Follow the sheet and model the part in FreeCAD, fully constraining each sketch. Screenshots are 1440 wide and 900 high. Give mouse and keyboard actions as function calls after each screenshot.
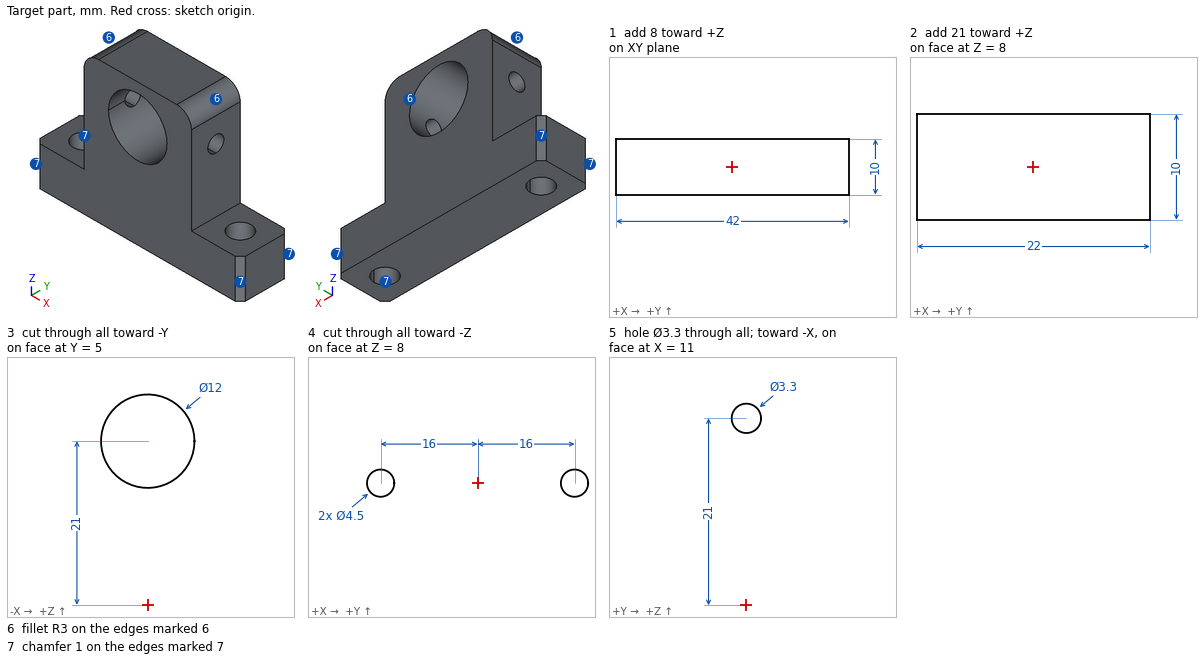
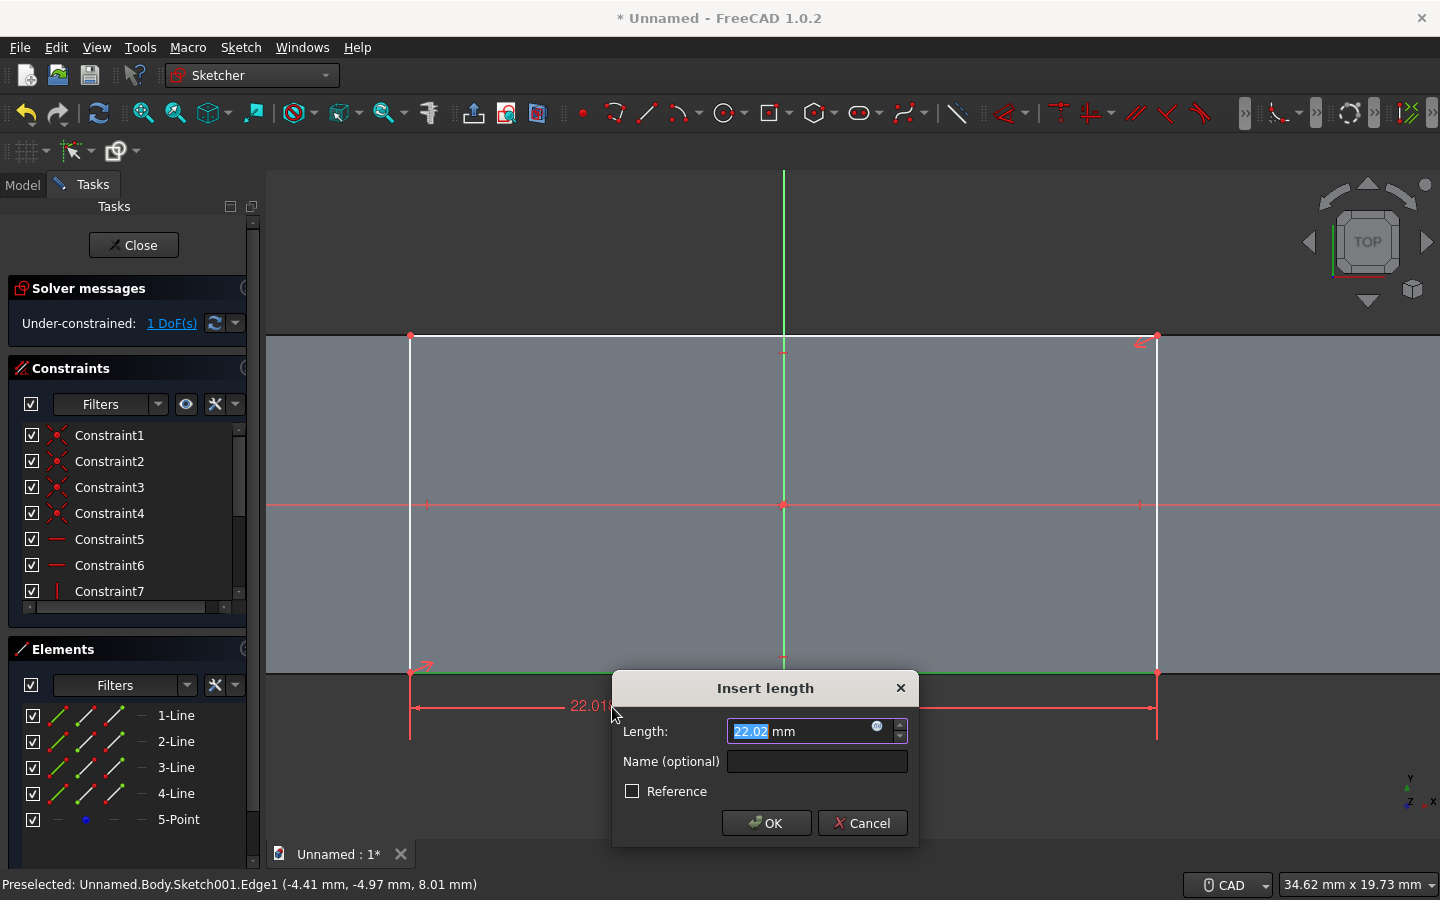
text(22)
key(Return)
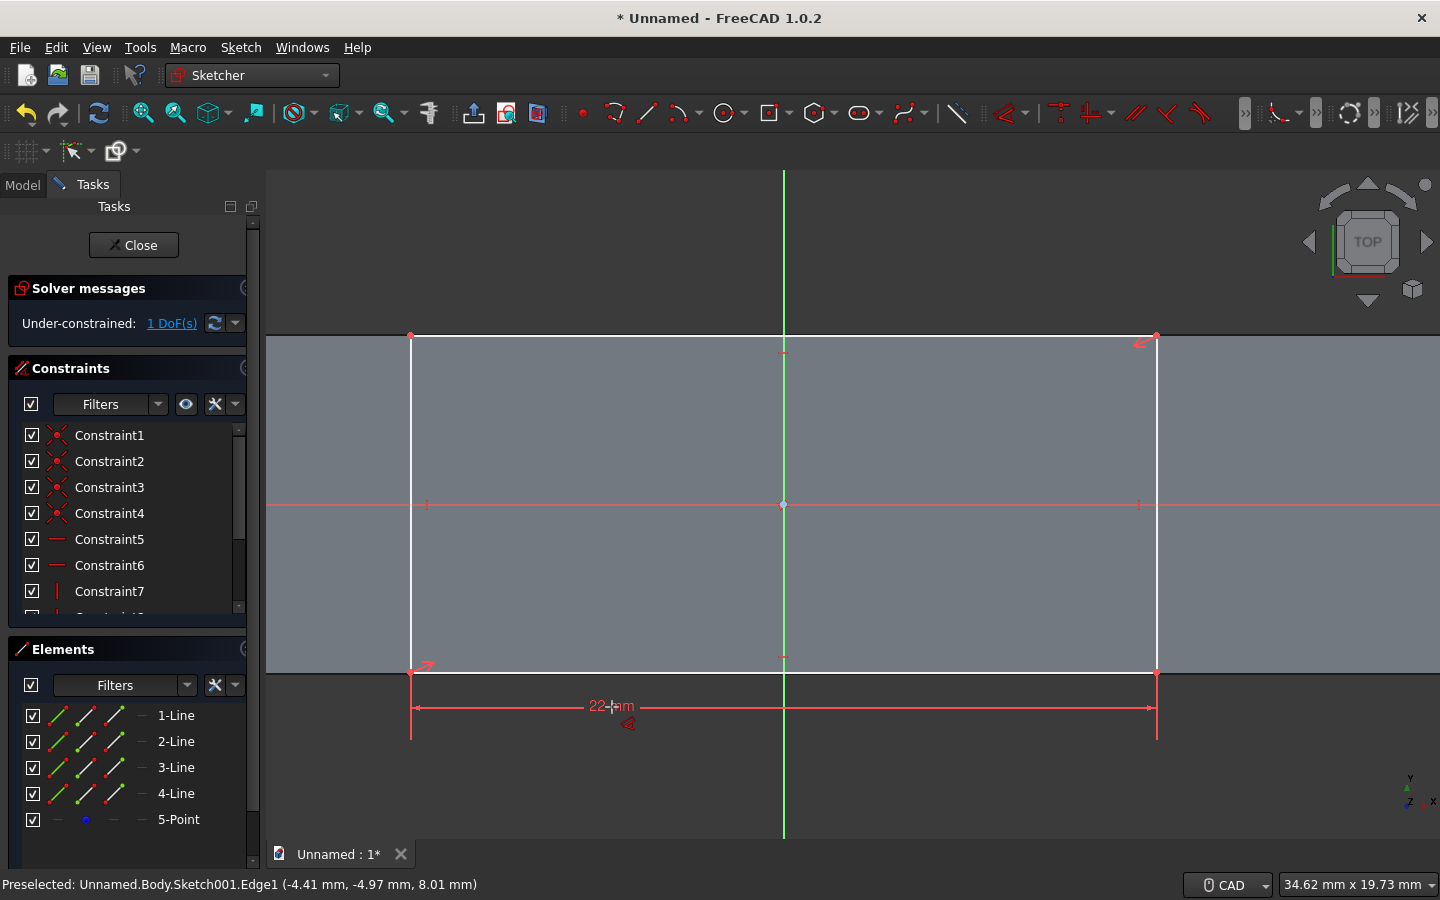
click(1157, 572)
click(1191, 427)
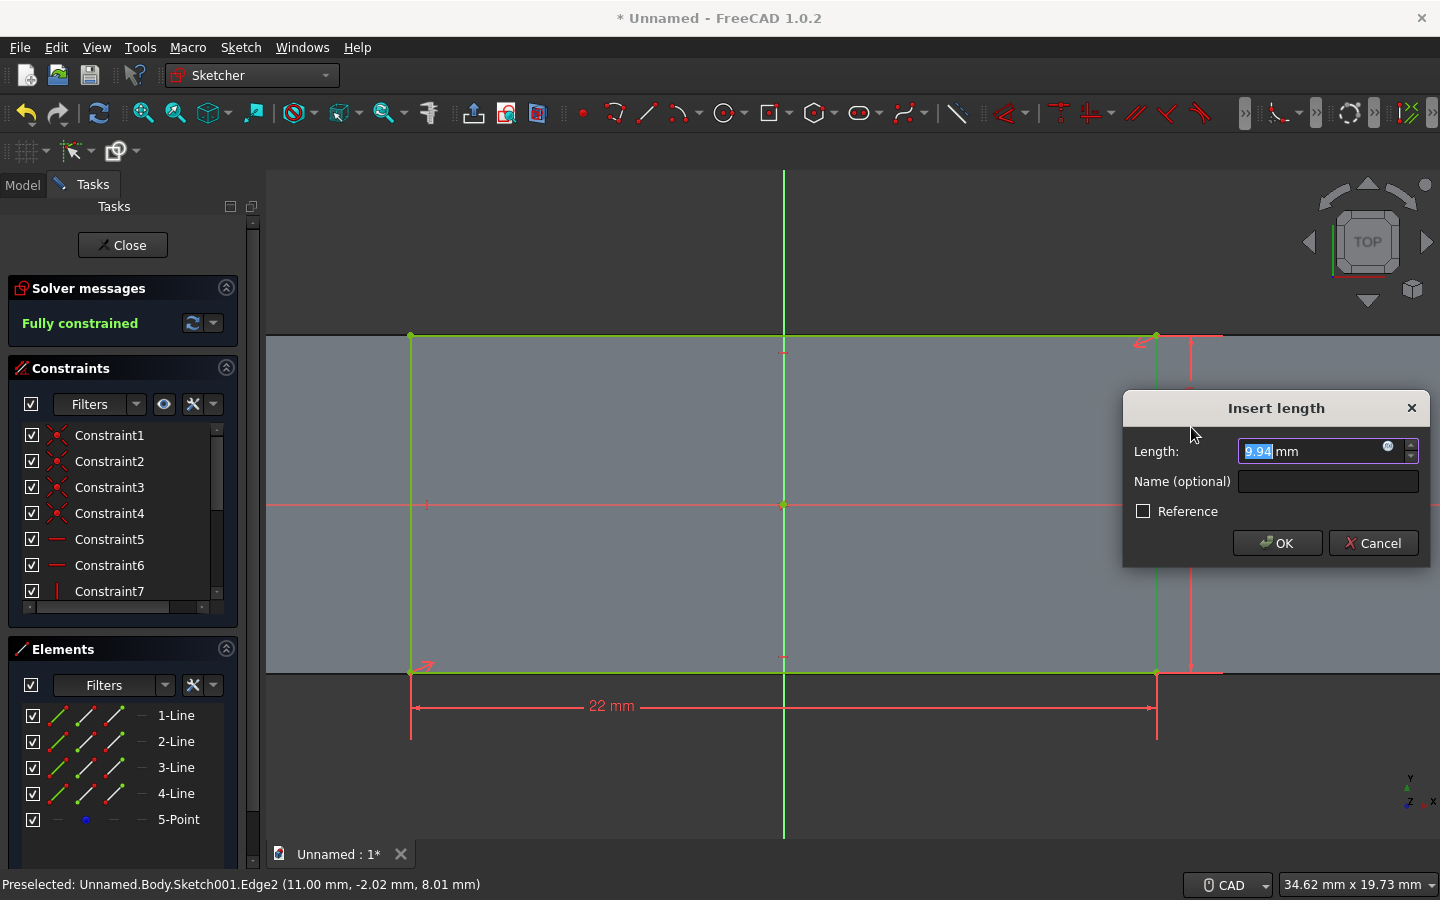
text(10)
key(Return)
key(Escape)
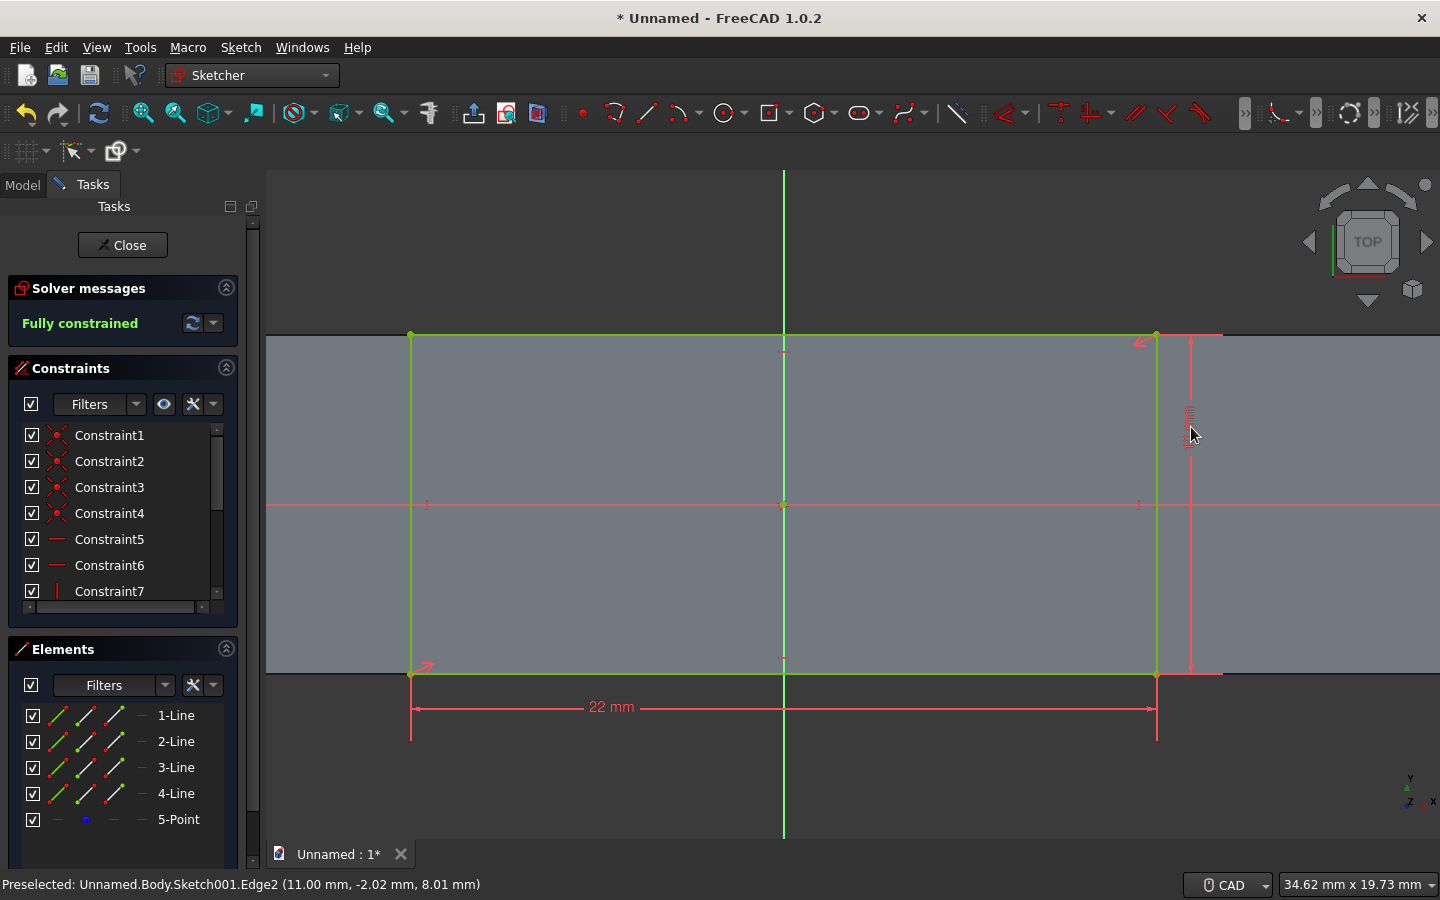
click(123, 245)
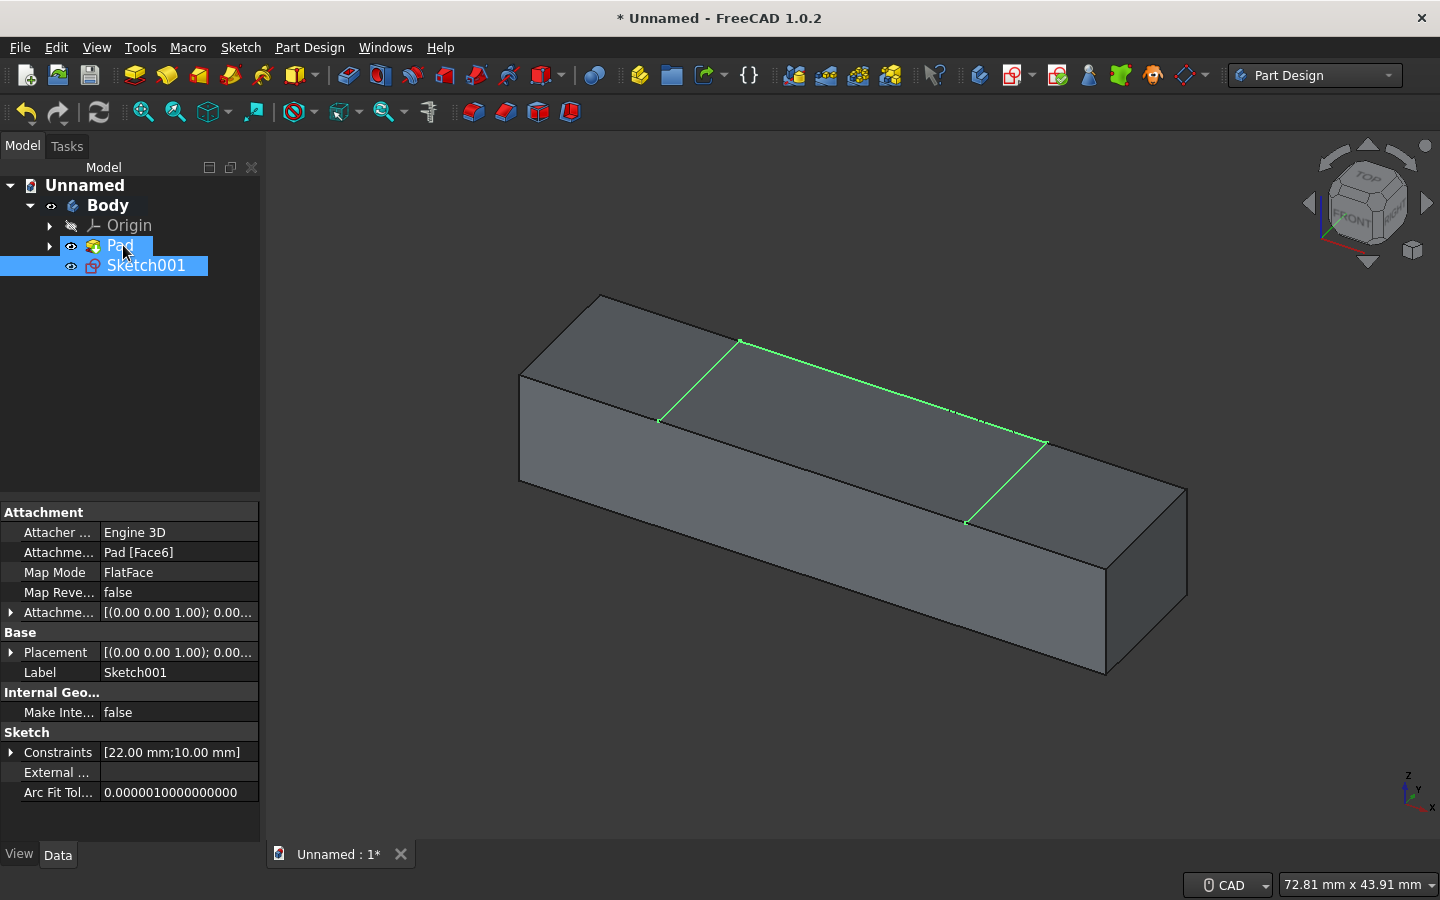
click(136, 76)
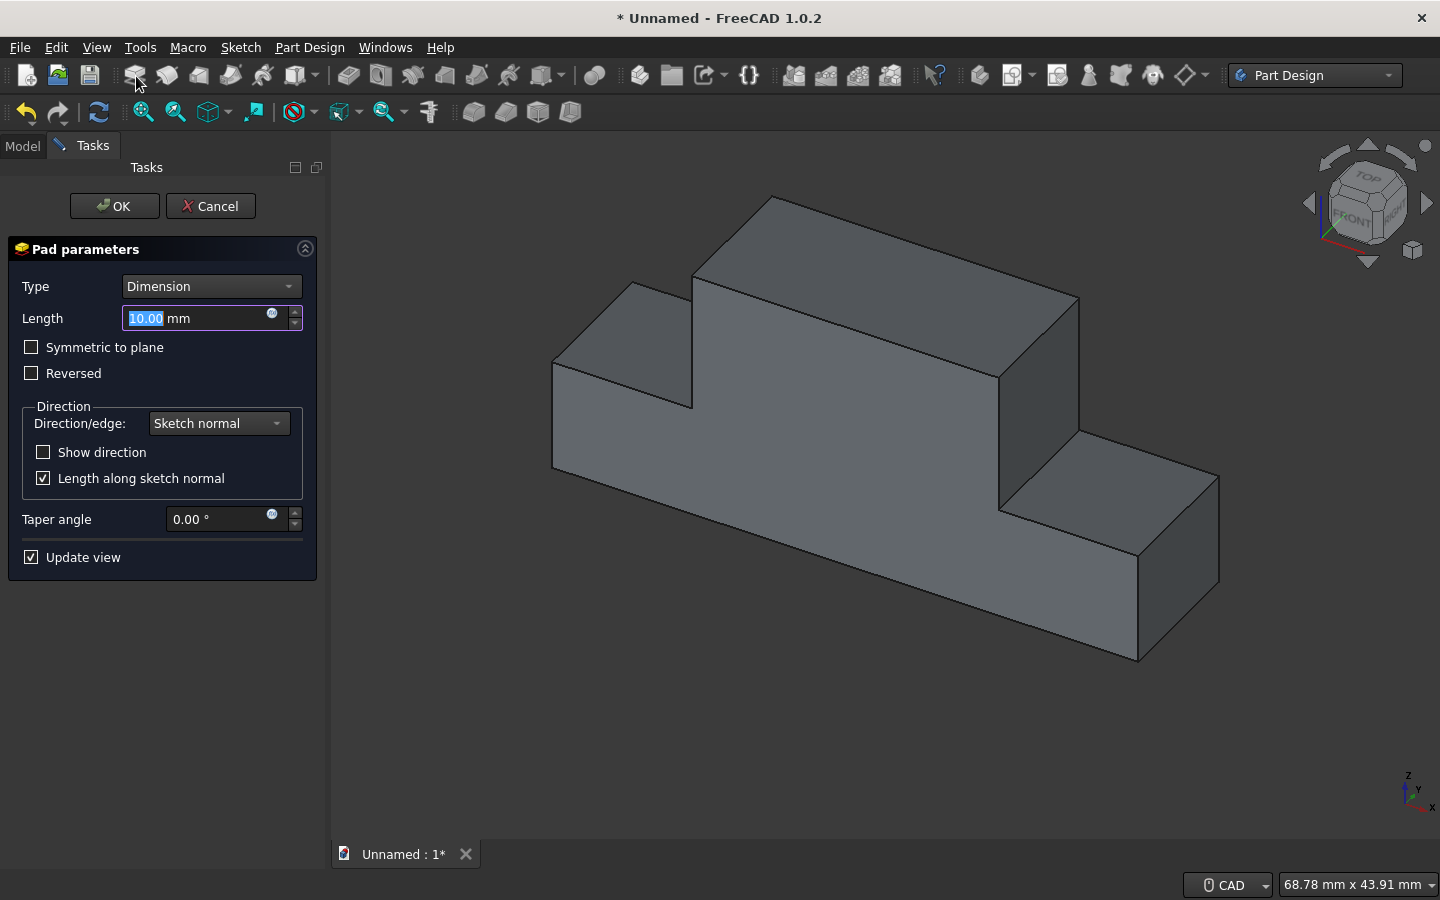
text(21)
key(Tab)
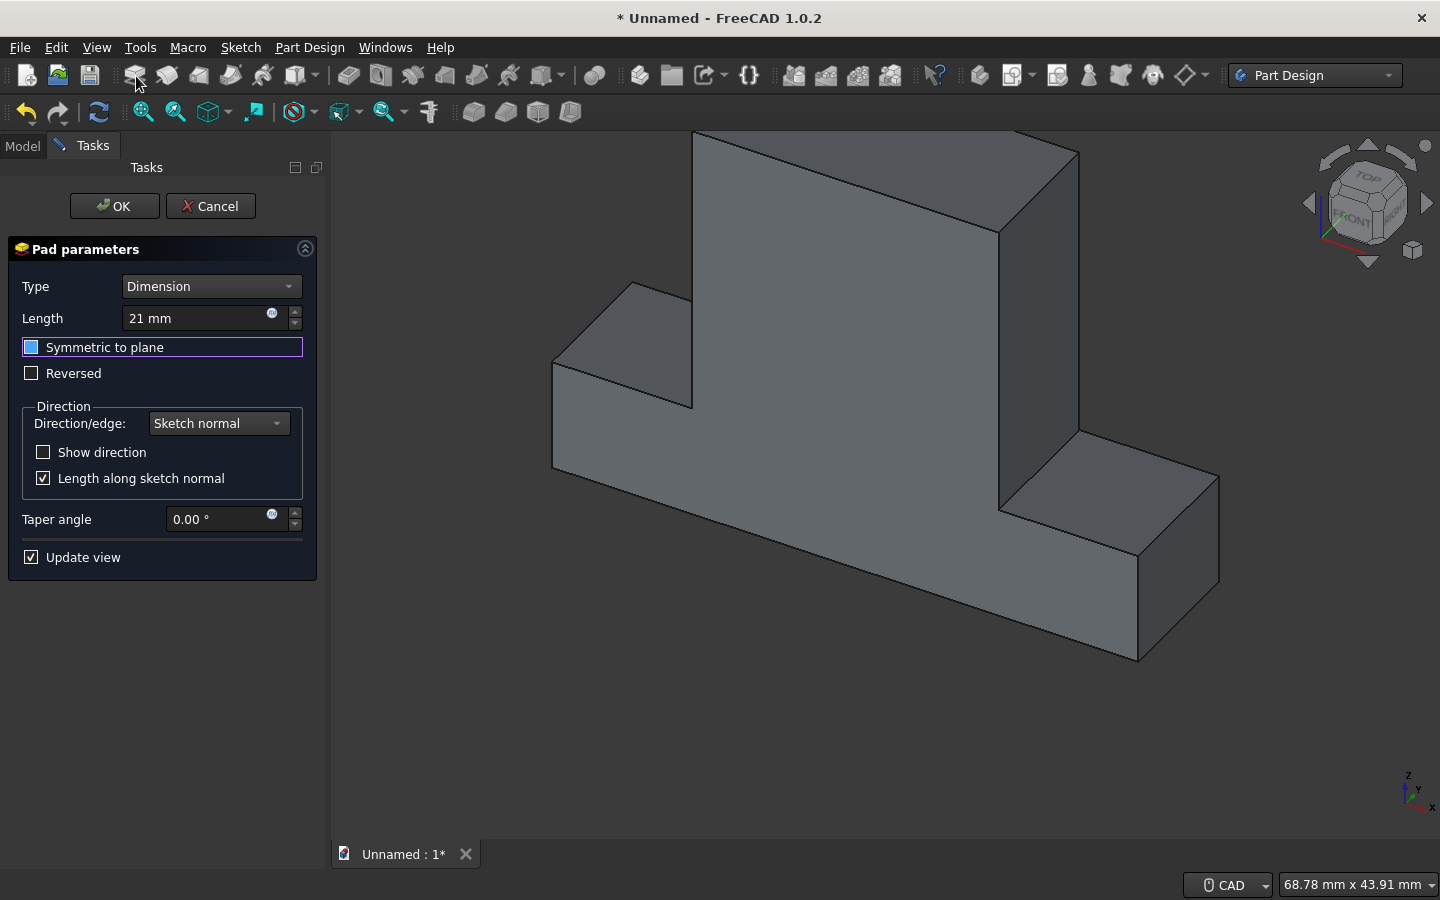
click(115, 206)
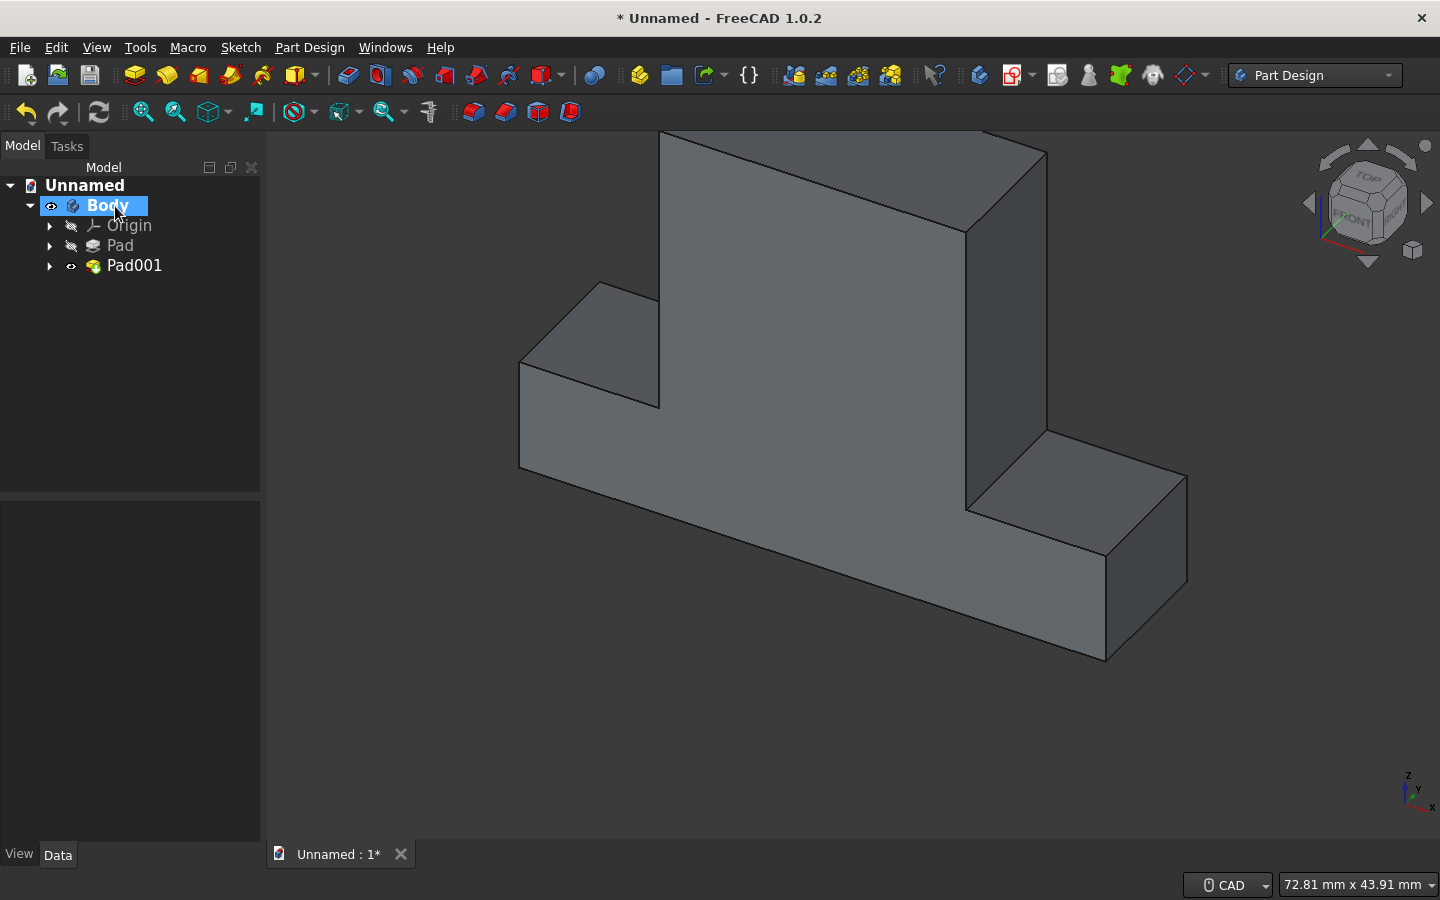
key(v)
key(f)